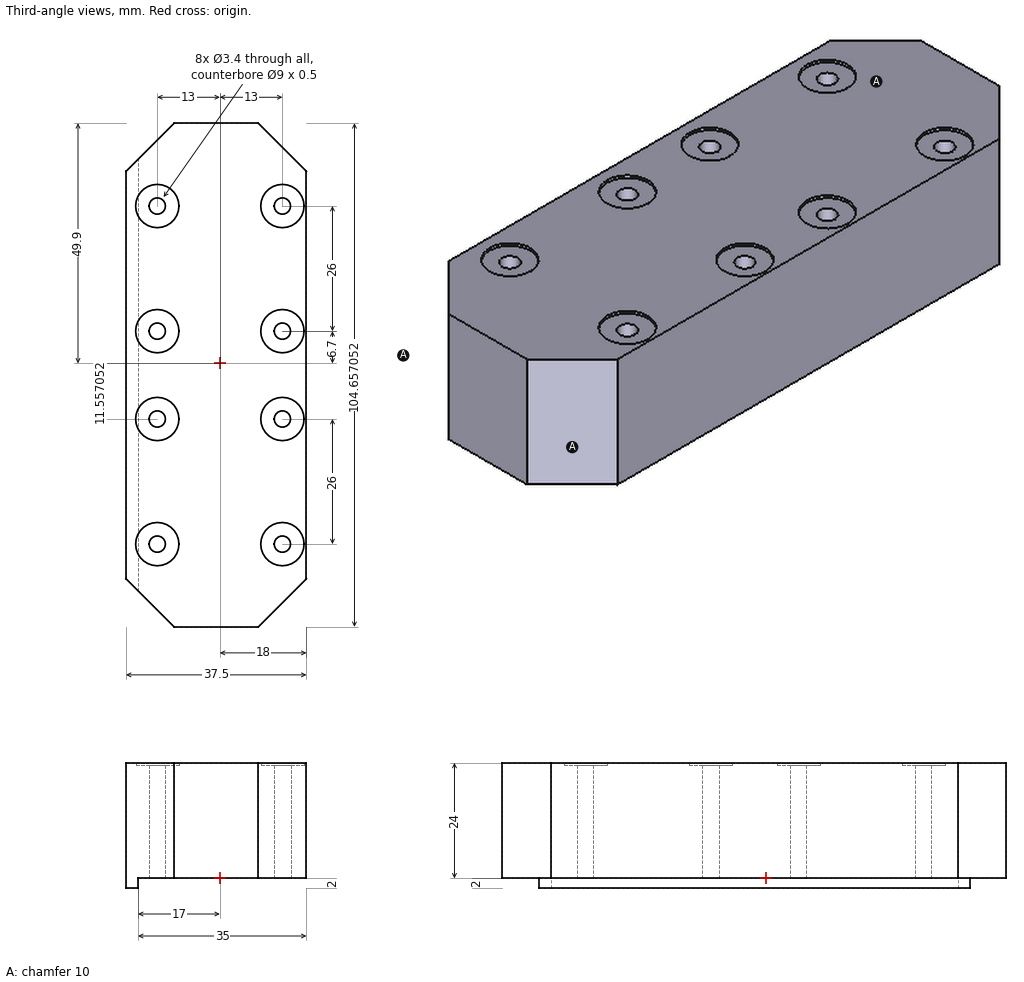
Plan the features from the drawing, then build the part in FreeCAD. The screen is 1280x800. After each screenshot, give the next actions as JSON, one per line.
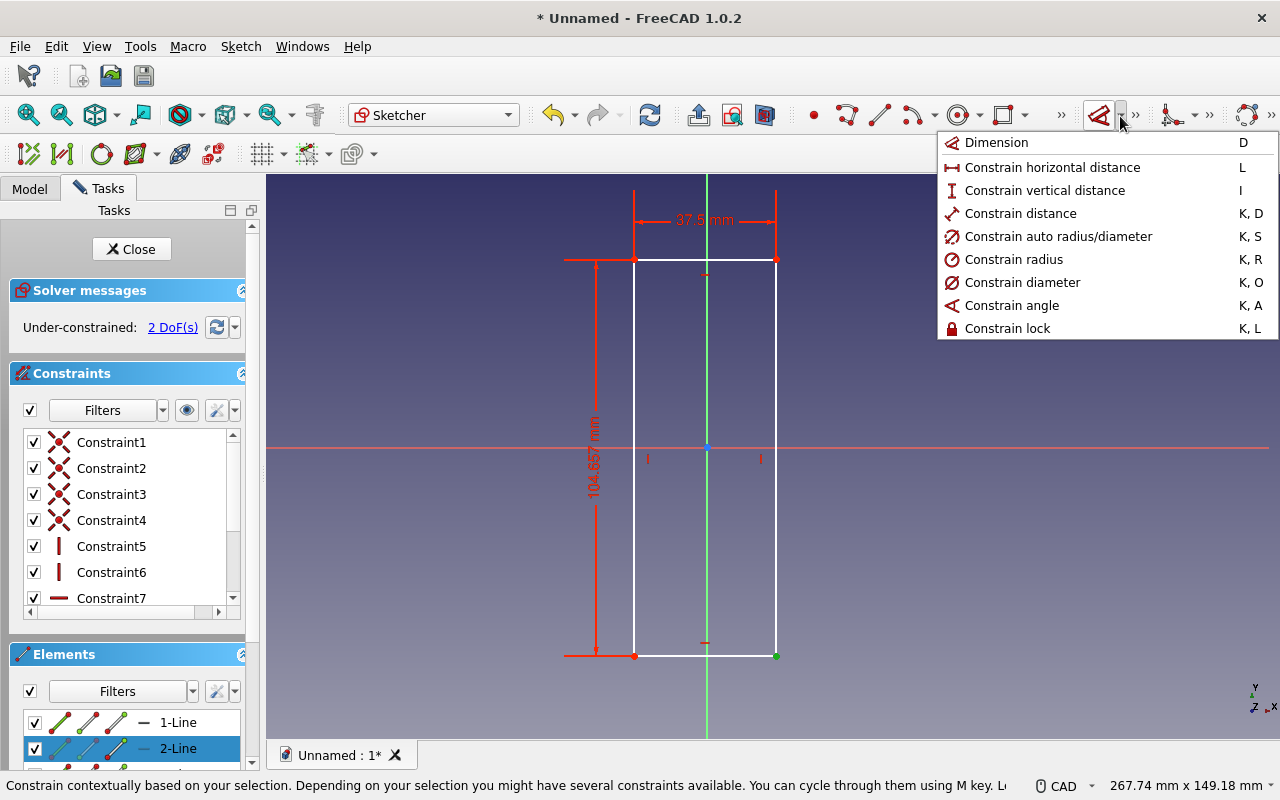
{"action": "left_click", "coordinate": [1108, 168]}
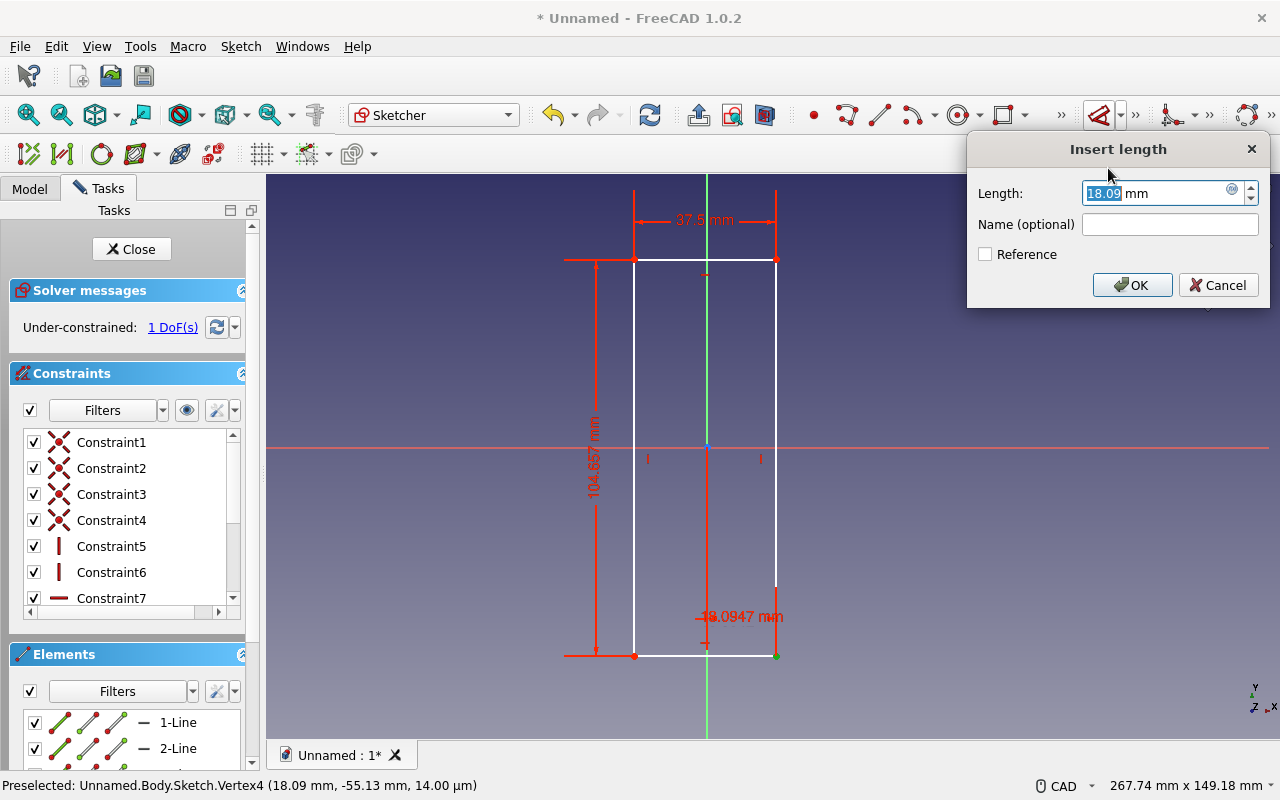
{"action": "type", "text": "18"}
{"action": "key", "text": "Return"}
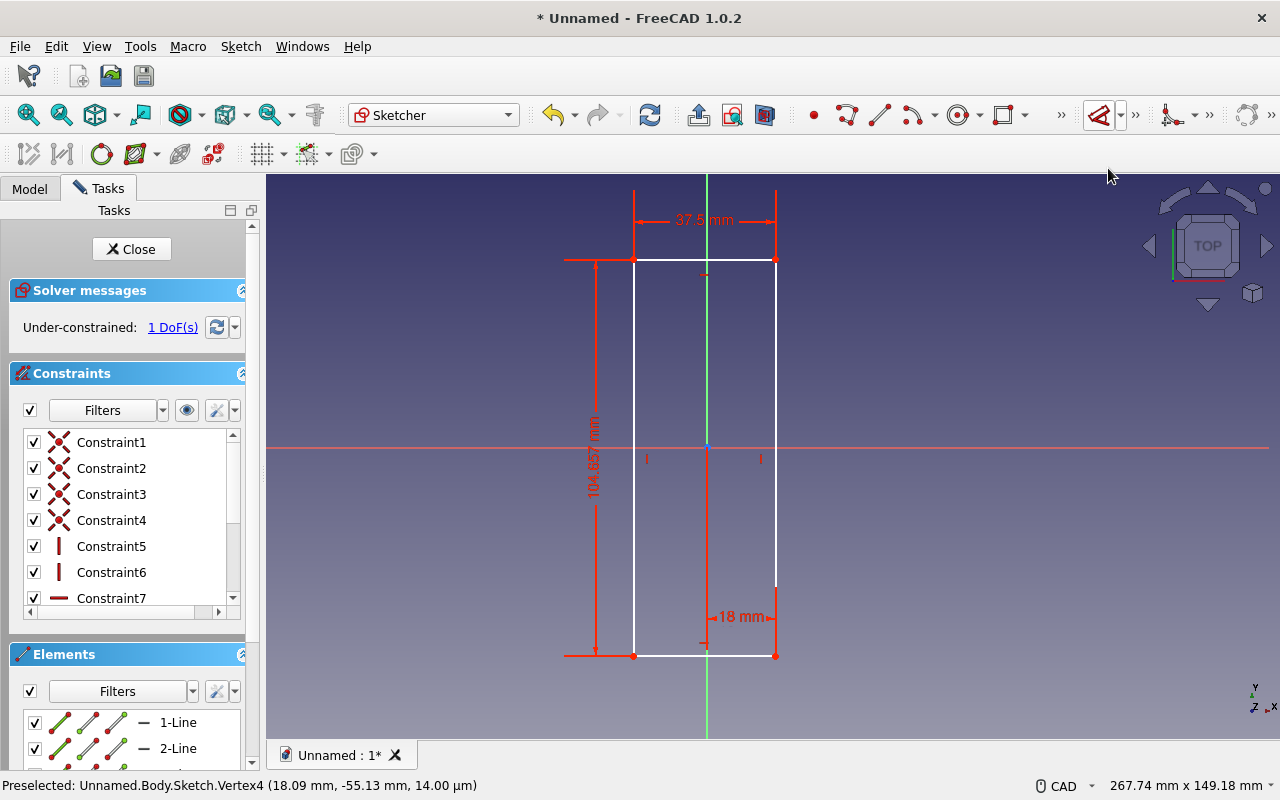
{"action": "left_click", "coordinate": [634, 260]}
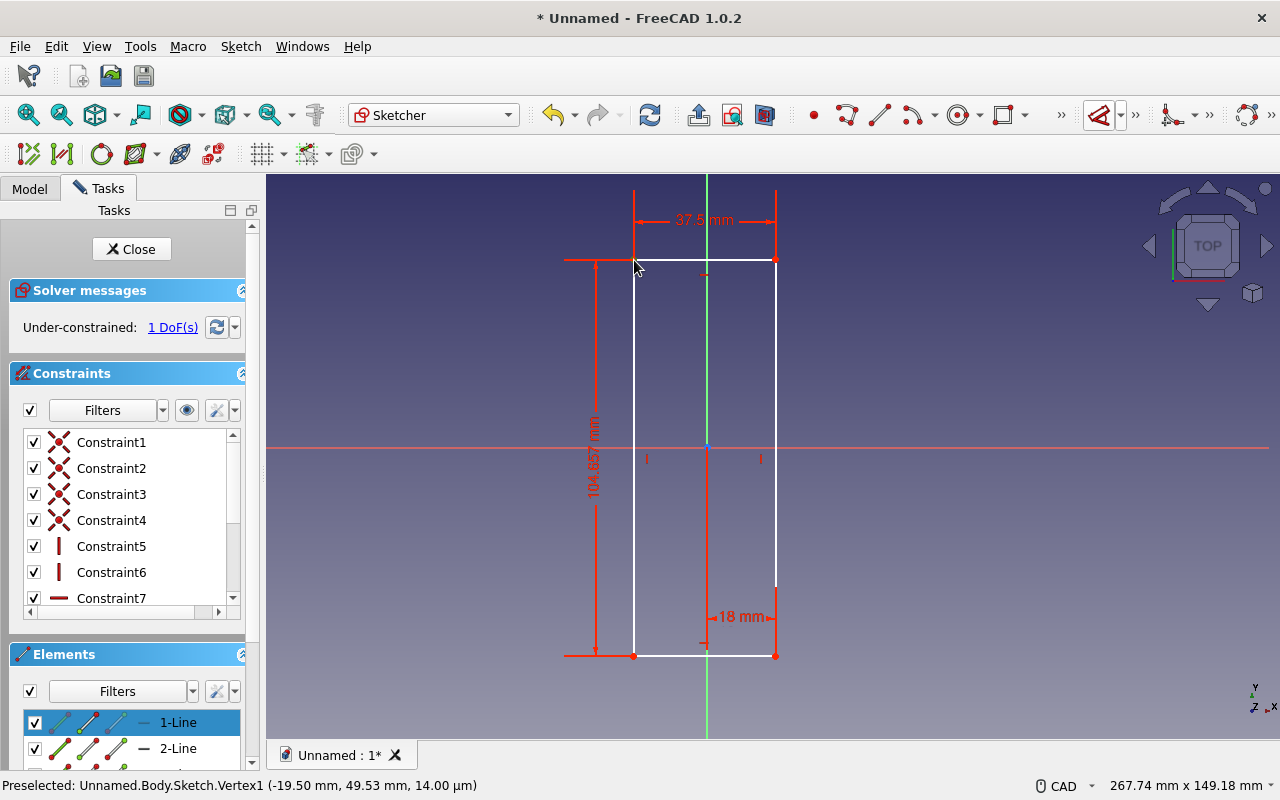
{"action": "left_click", "coordinate": [1120, 116]}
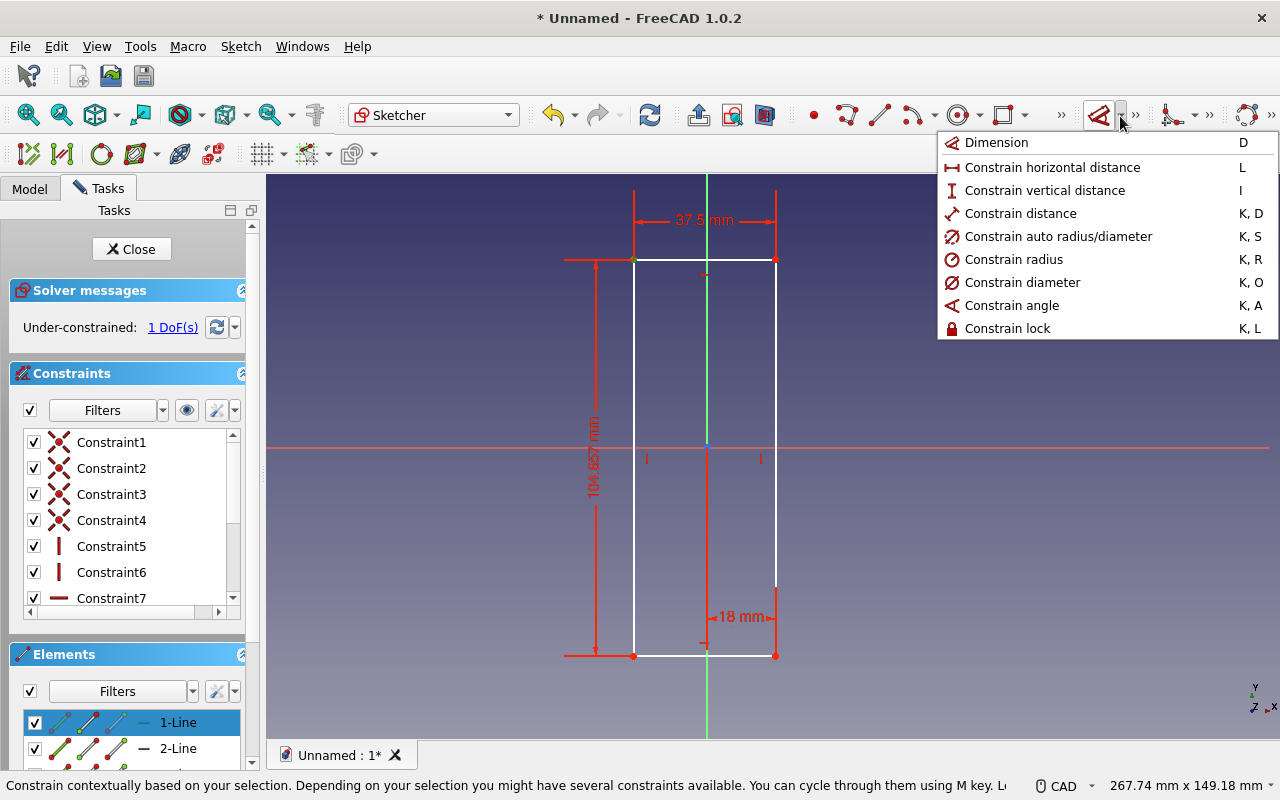
{"action": "left_click", "coordinate": [1108, 190]}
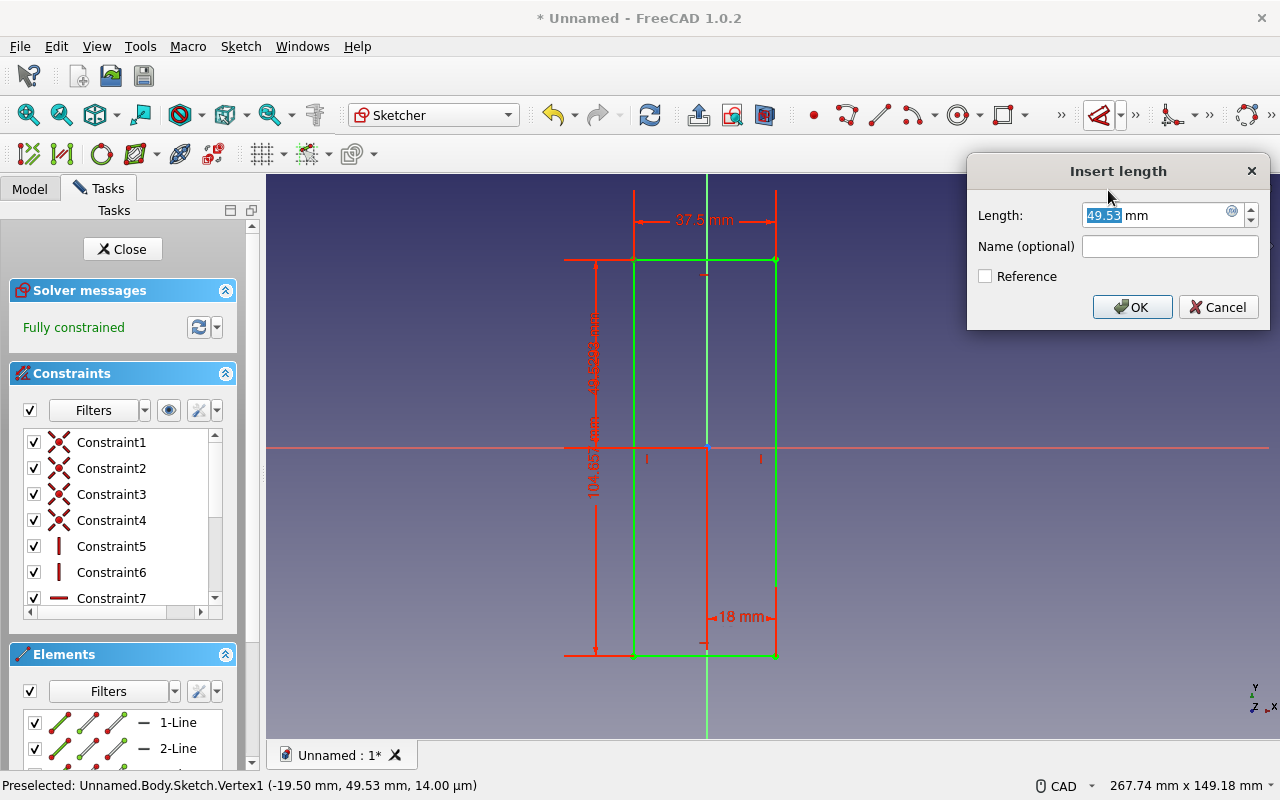
{"action": "type", "text": "49.9"}
{"action": "key", "text": "Return"}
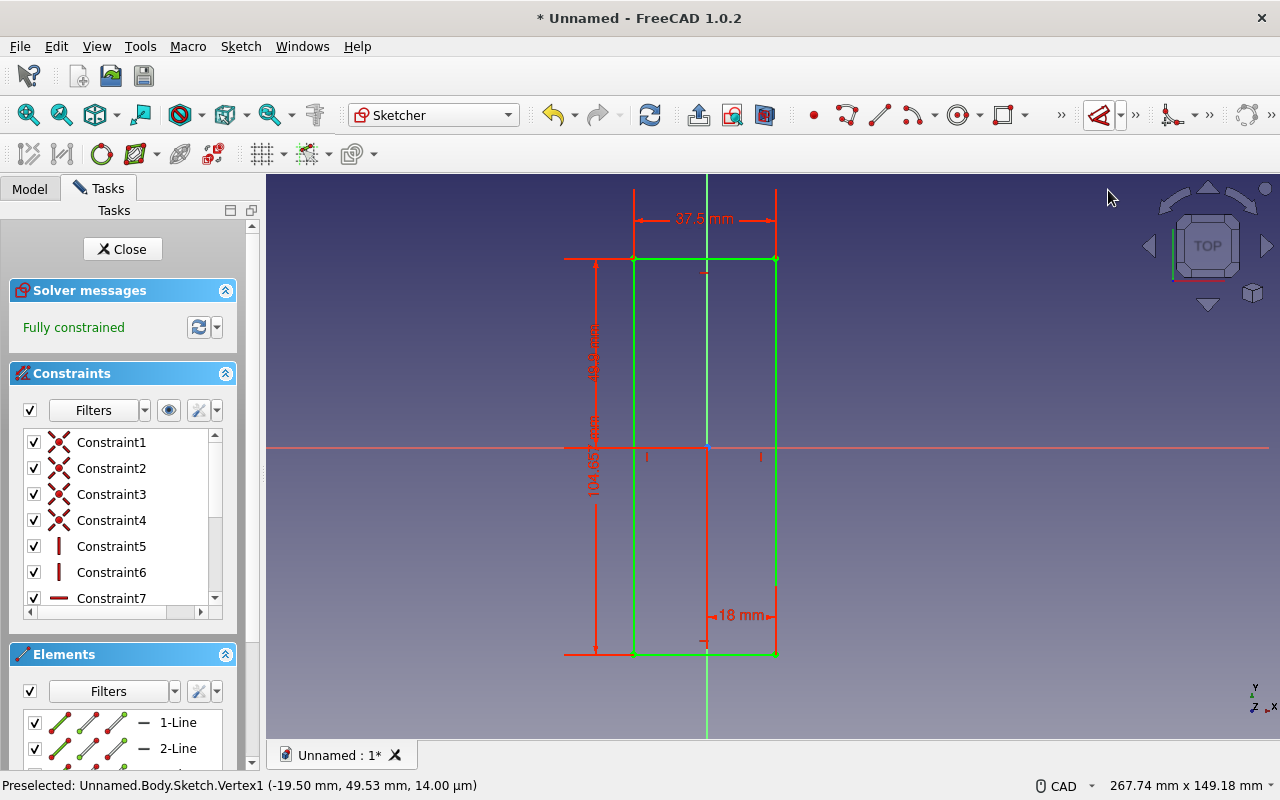
{"action": "left_click", "coordinate": [123, 249]}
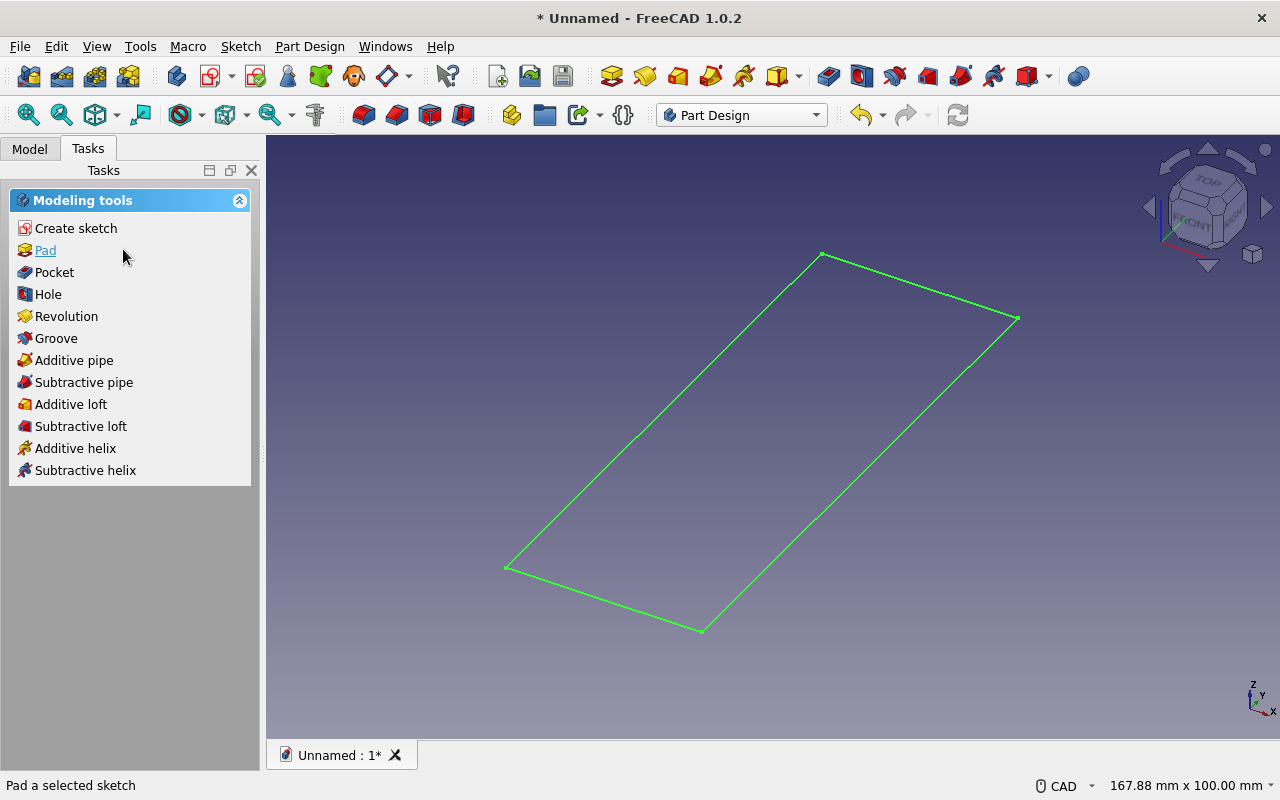
{"action": "left_click", "coordinate": [612, 76]}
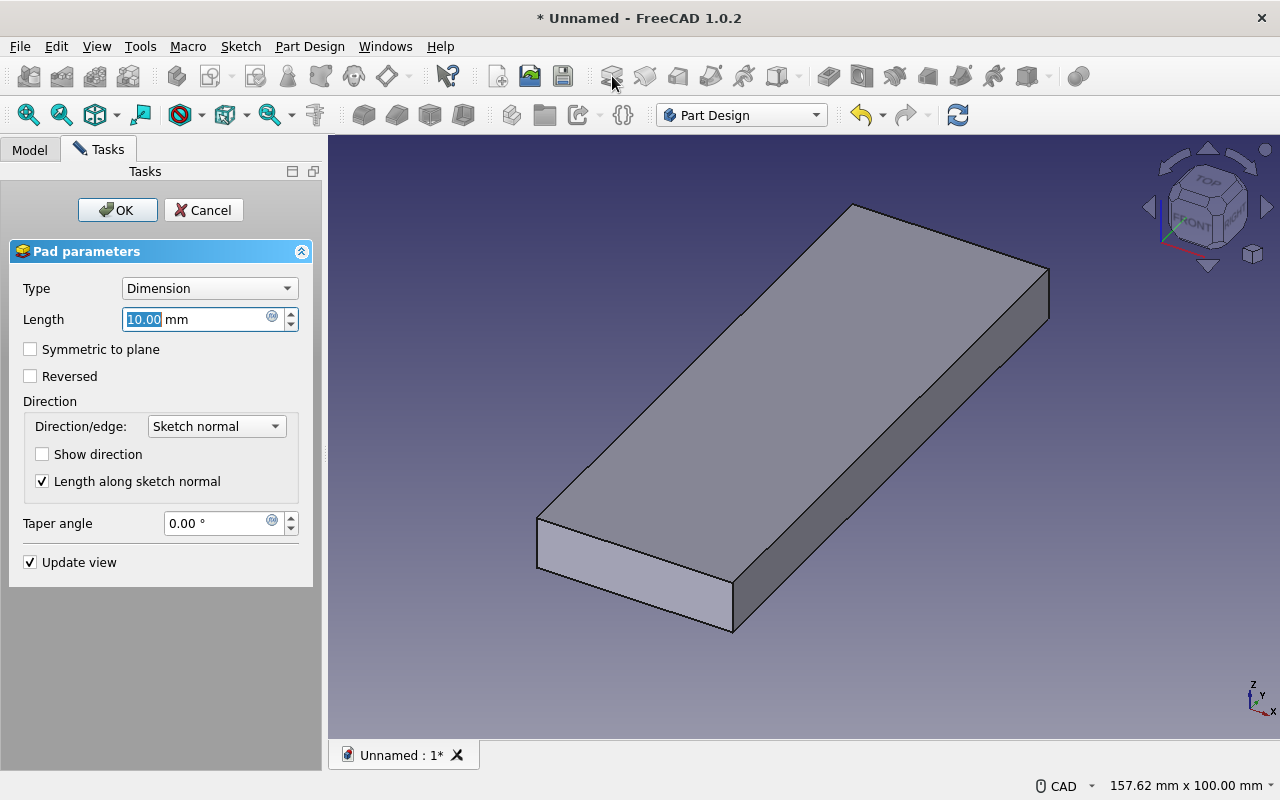
{"action": "left_click", "coordinate": [210, 288]}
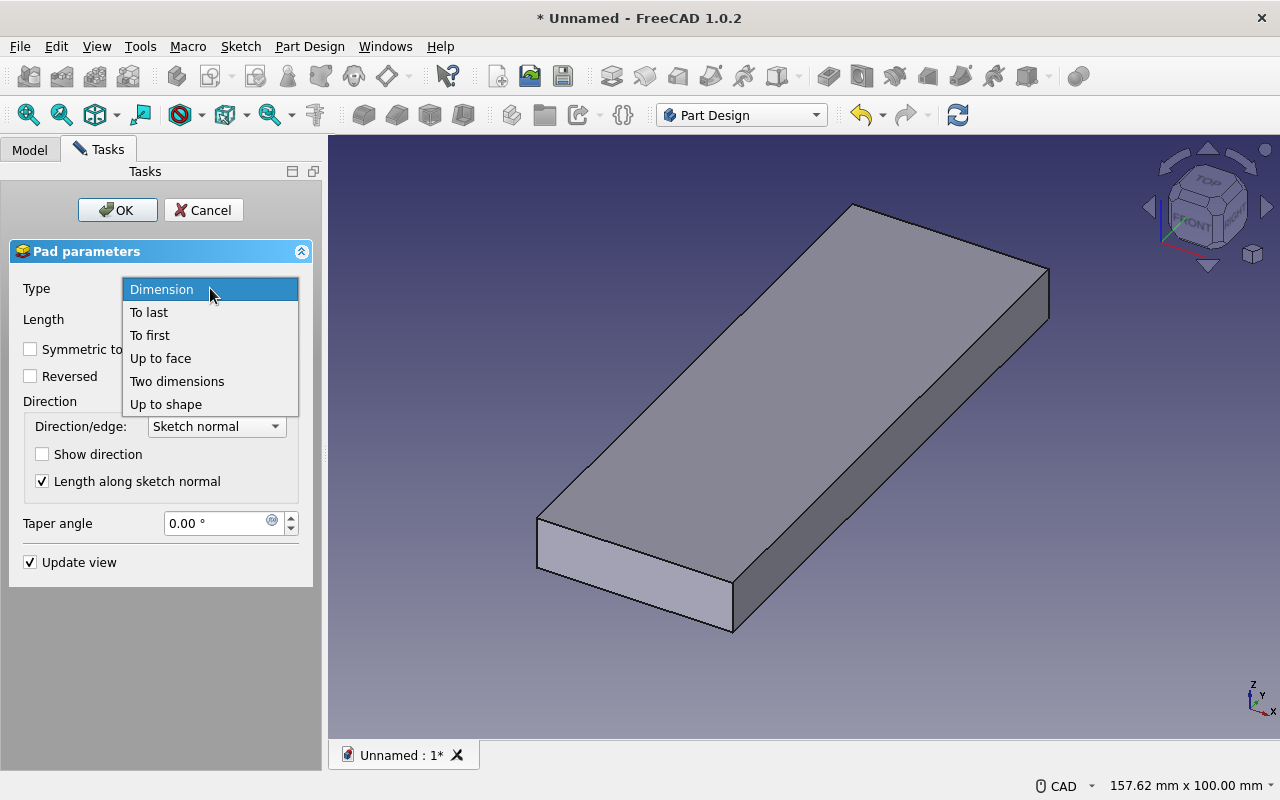
{"action": "left_click", "coordinate": [208, 382]}